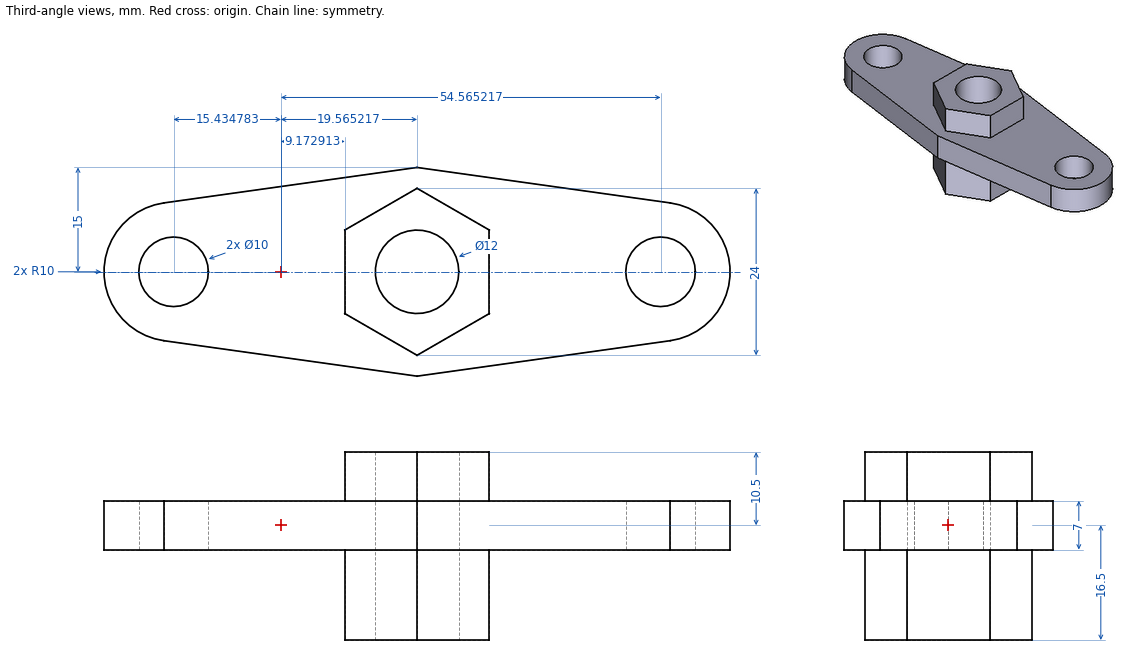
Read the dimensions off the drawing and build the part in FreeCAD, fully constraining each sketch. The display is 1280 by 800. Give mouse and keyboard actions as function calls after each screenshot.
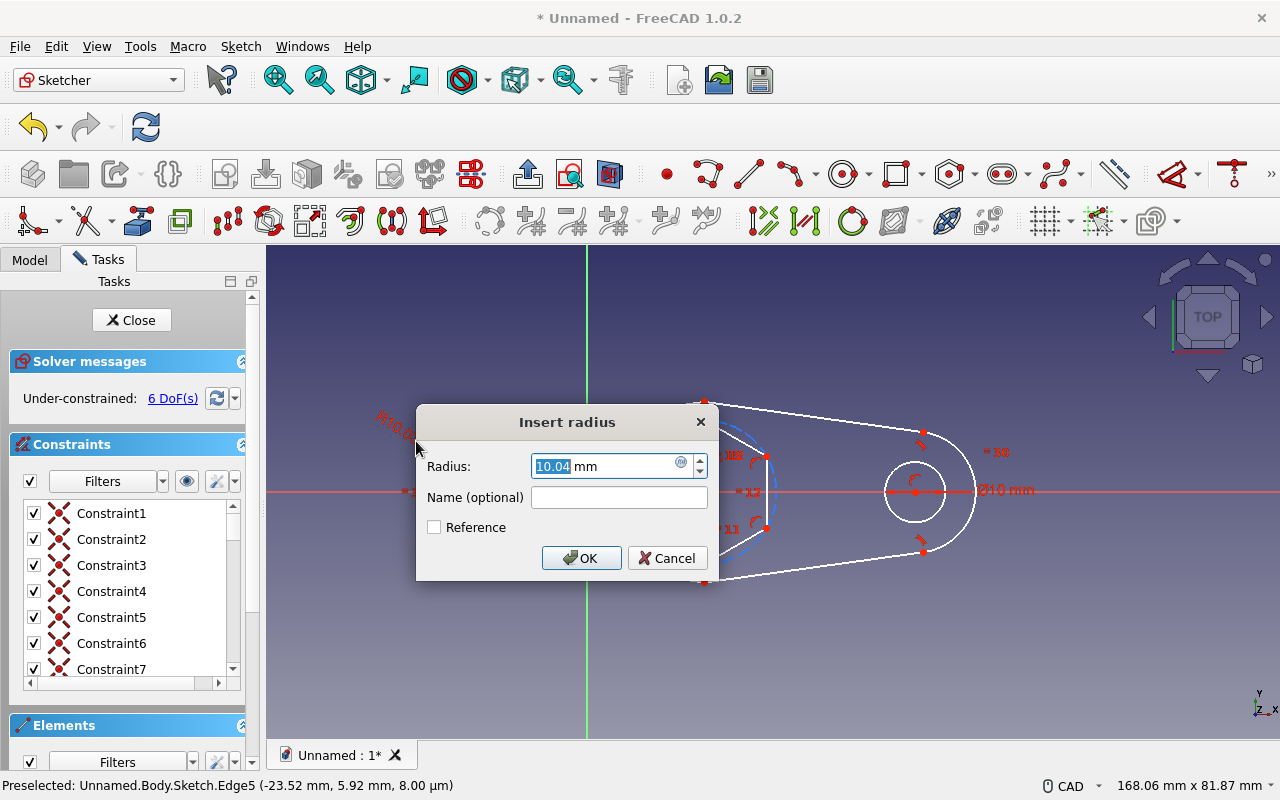
text(10)
key(Return)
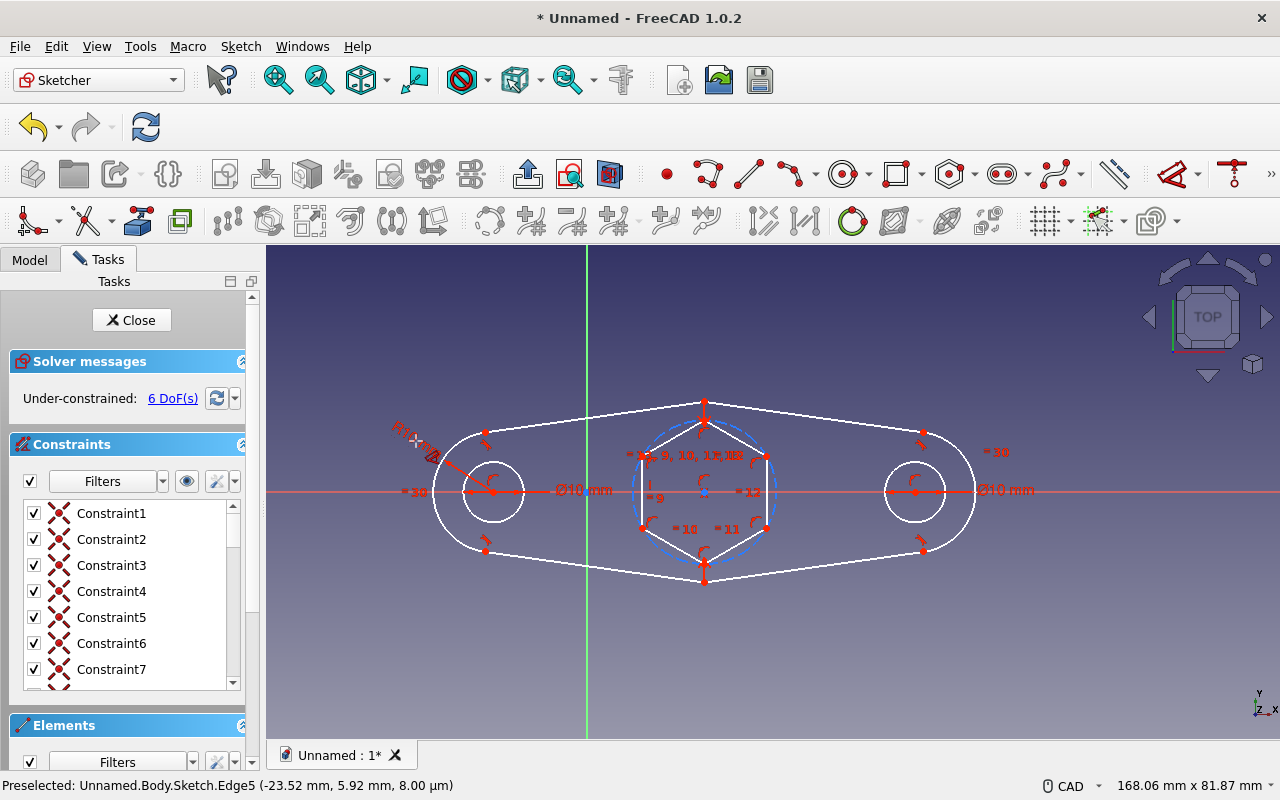
click(704, 564)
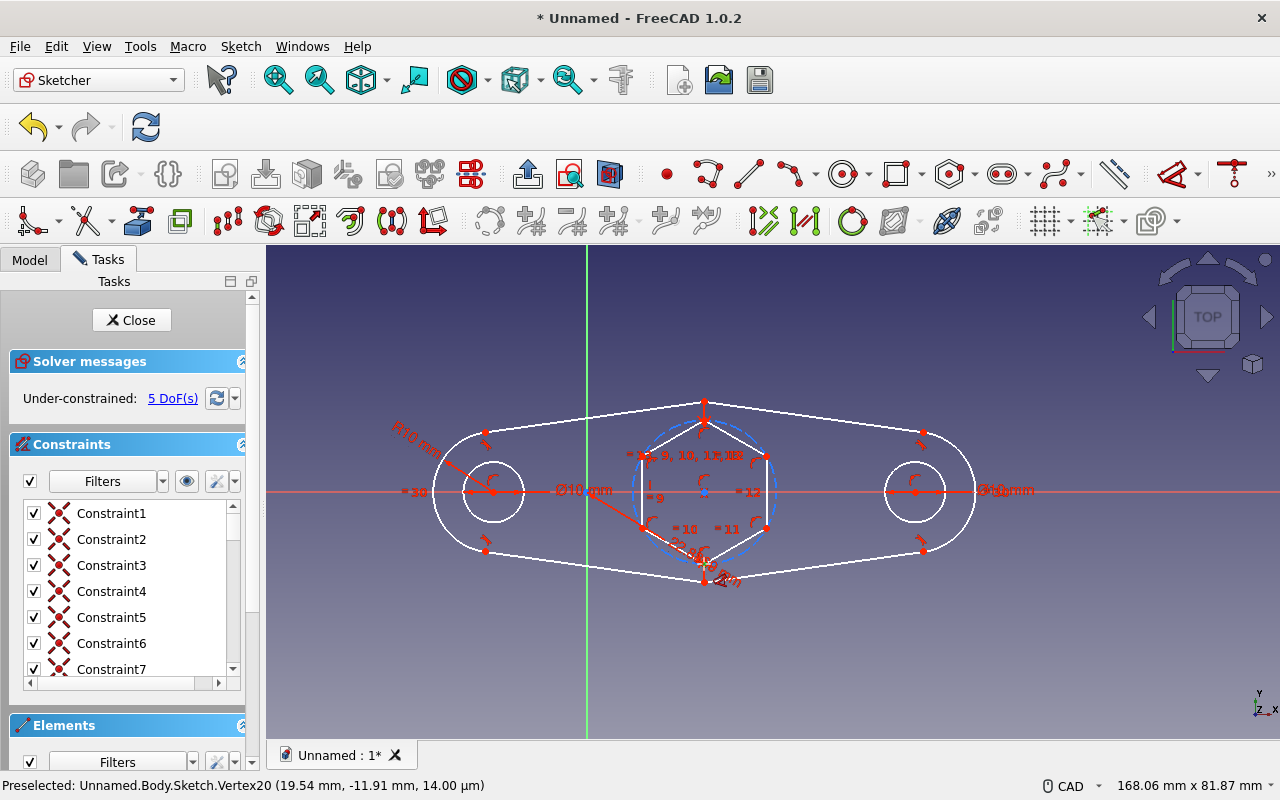
click(704, 420)
click(670, 459)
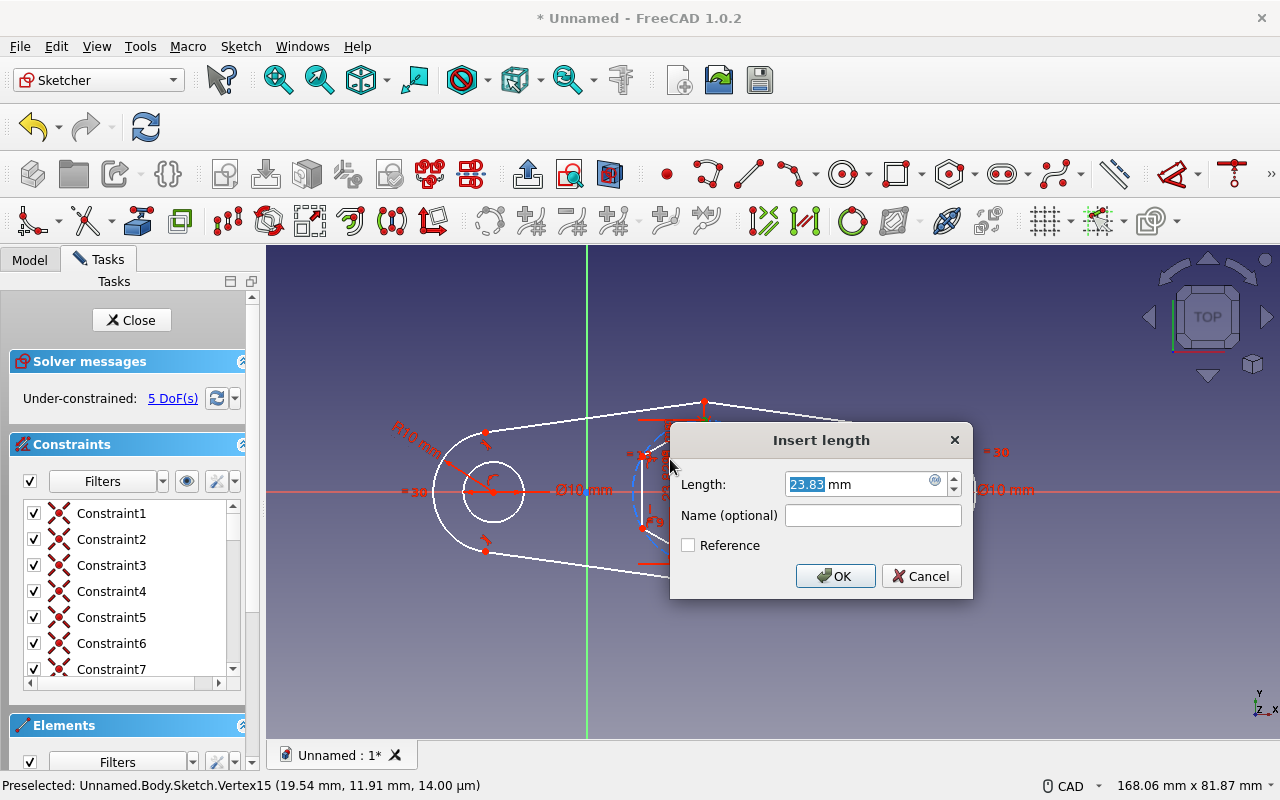
text(24)
key(Return)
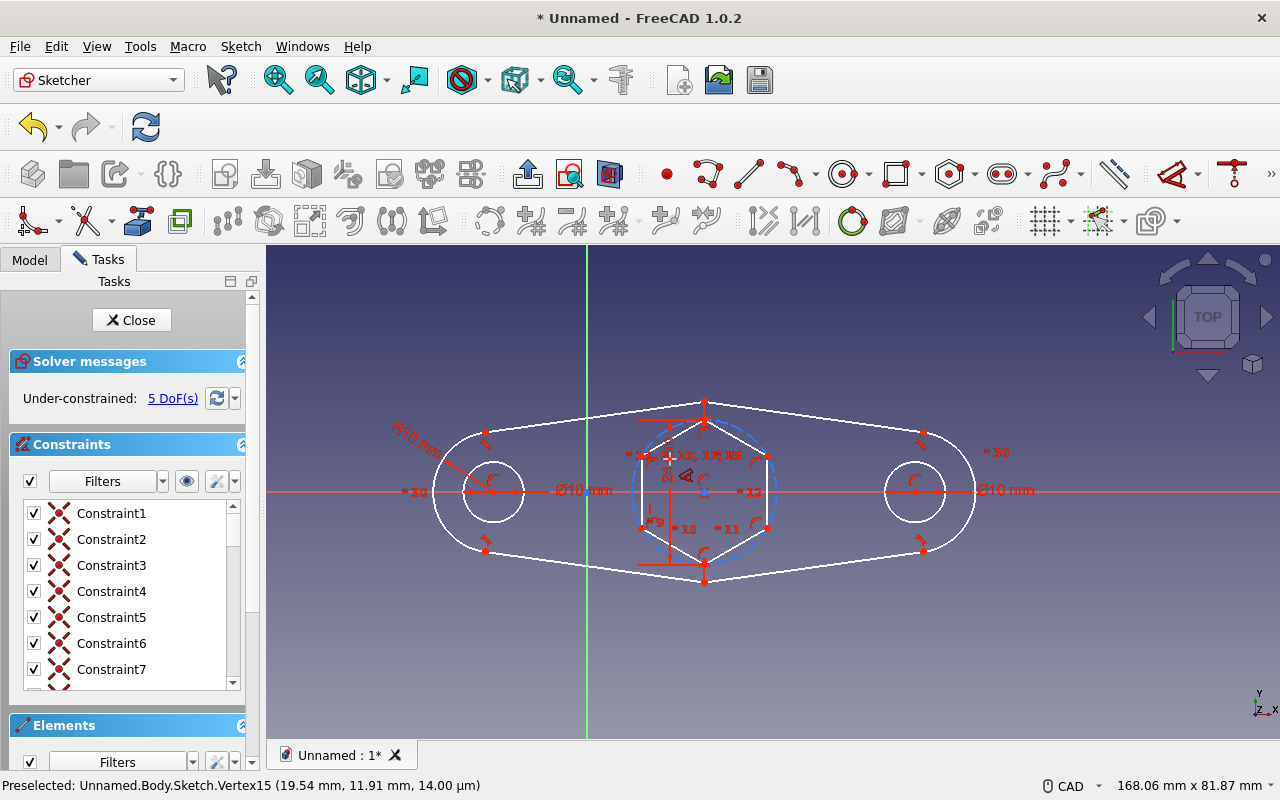
click(704, 402)
click(553, 447)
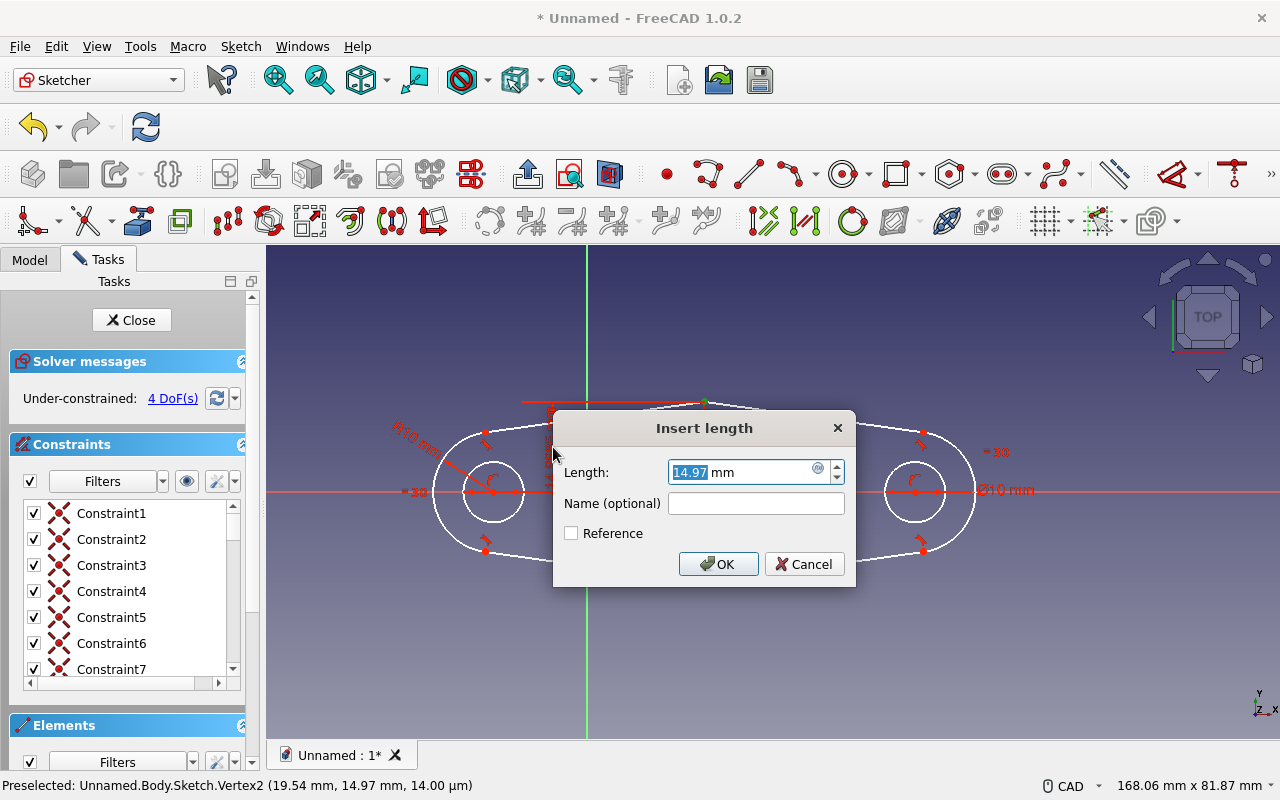
text(15)
key(Return)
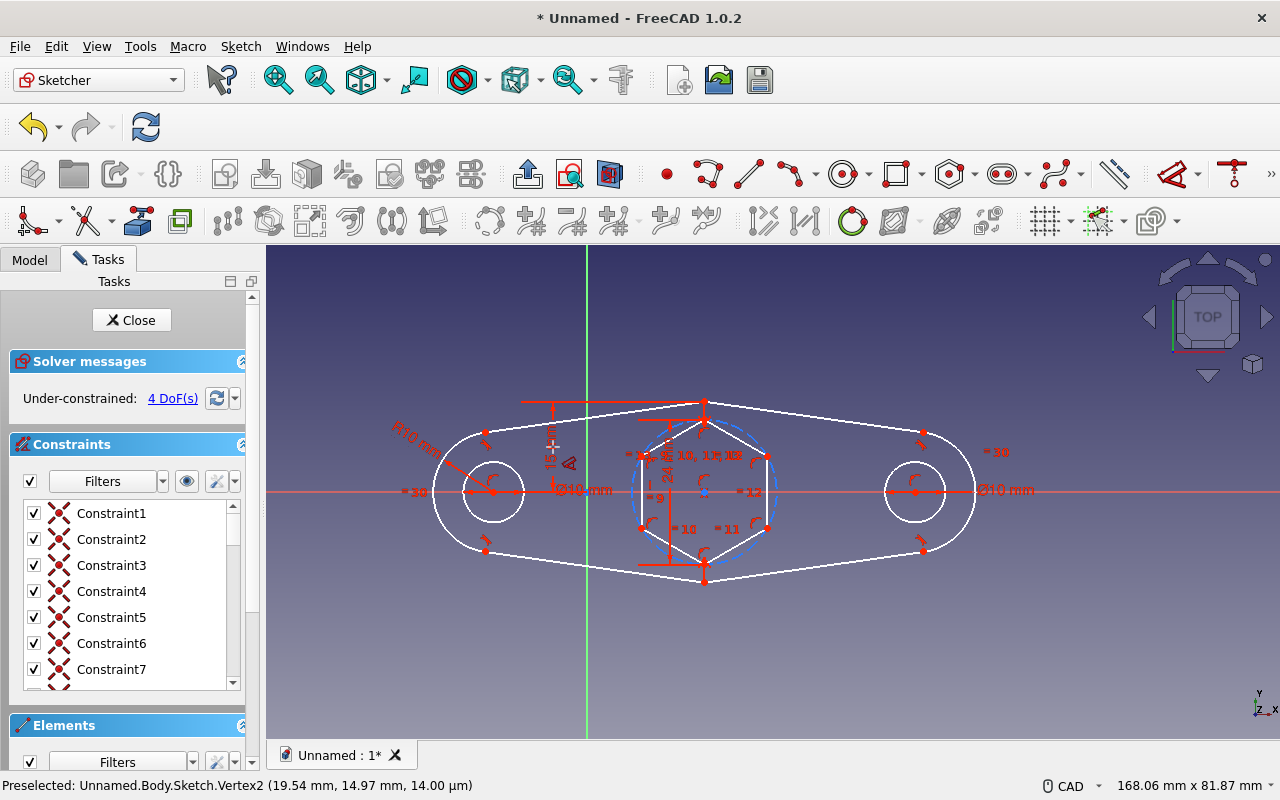
click(642, 456)
click(614, 526)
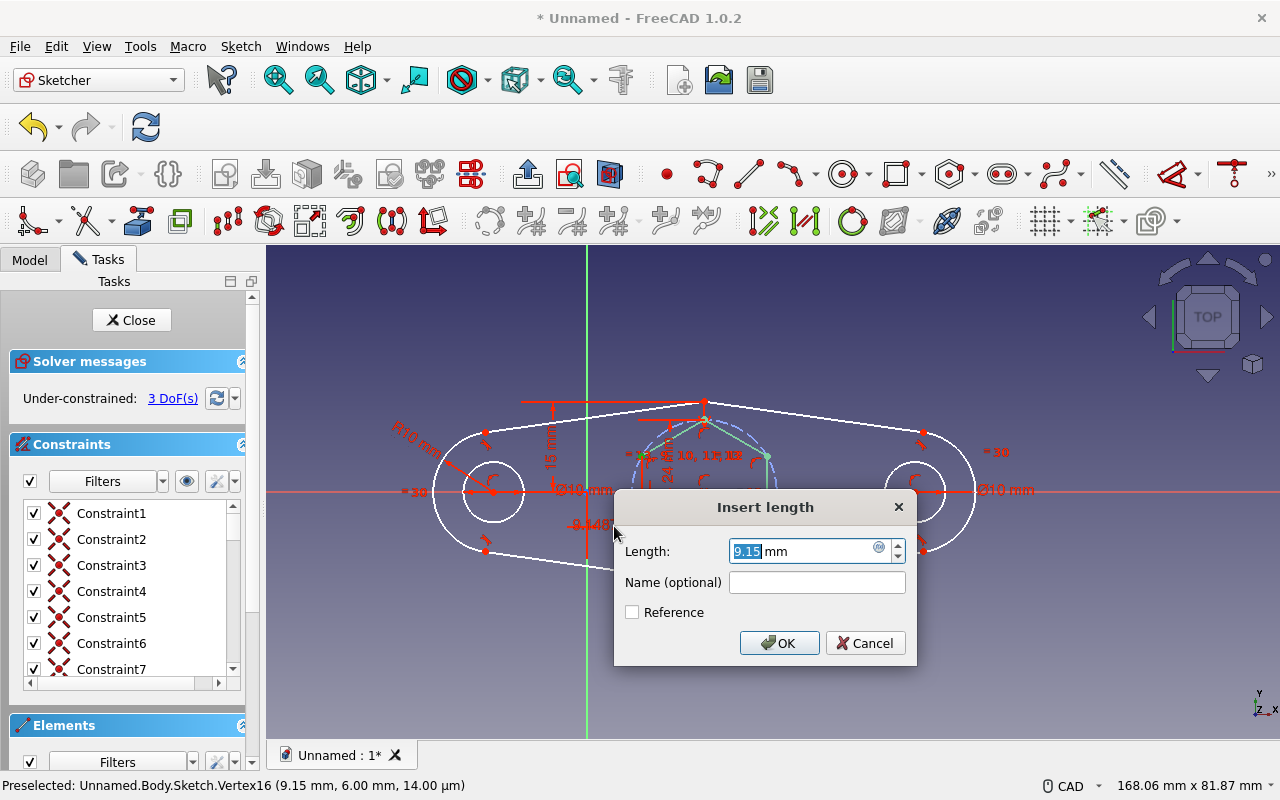
text(9.172913)
key(Return)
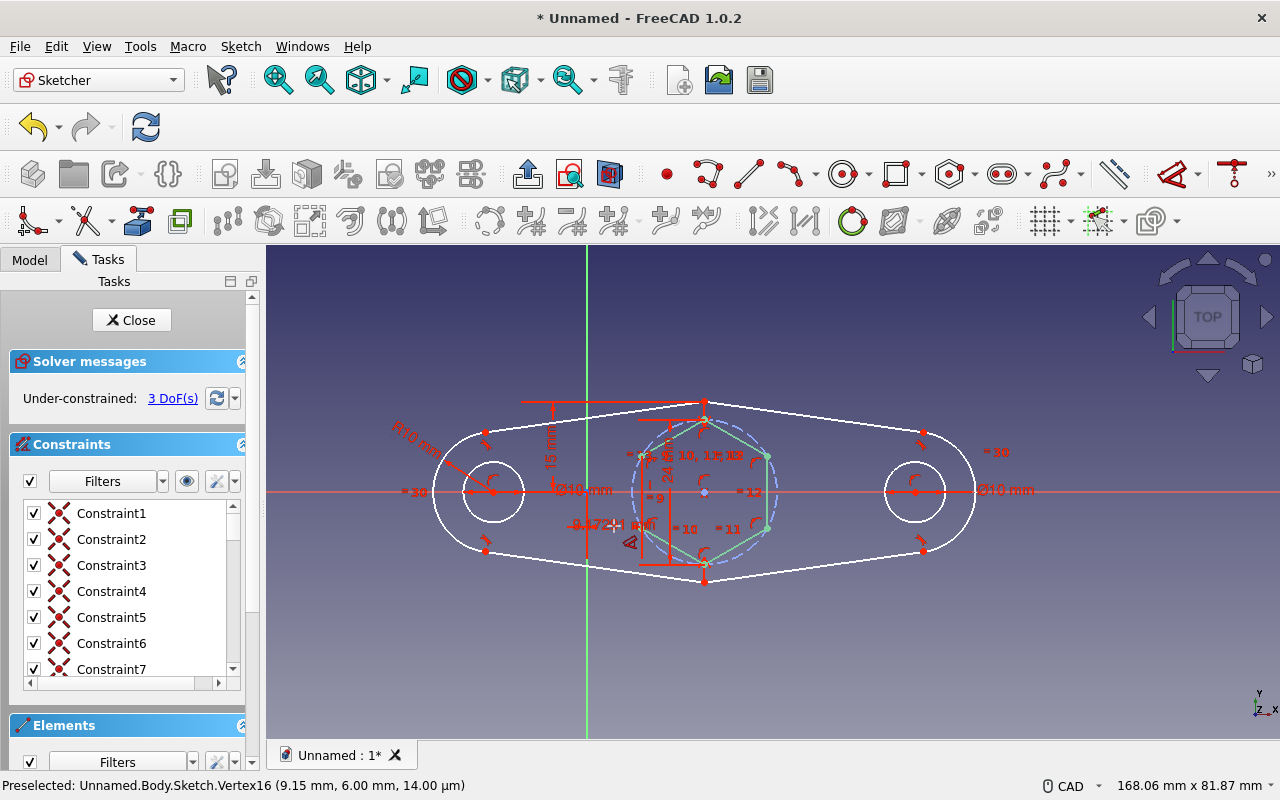
click(494, 492)
click(540, 526)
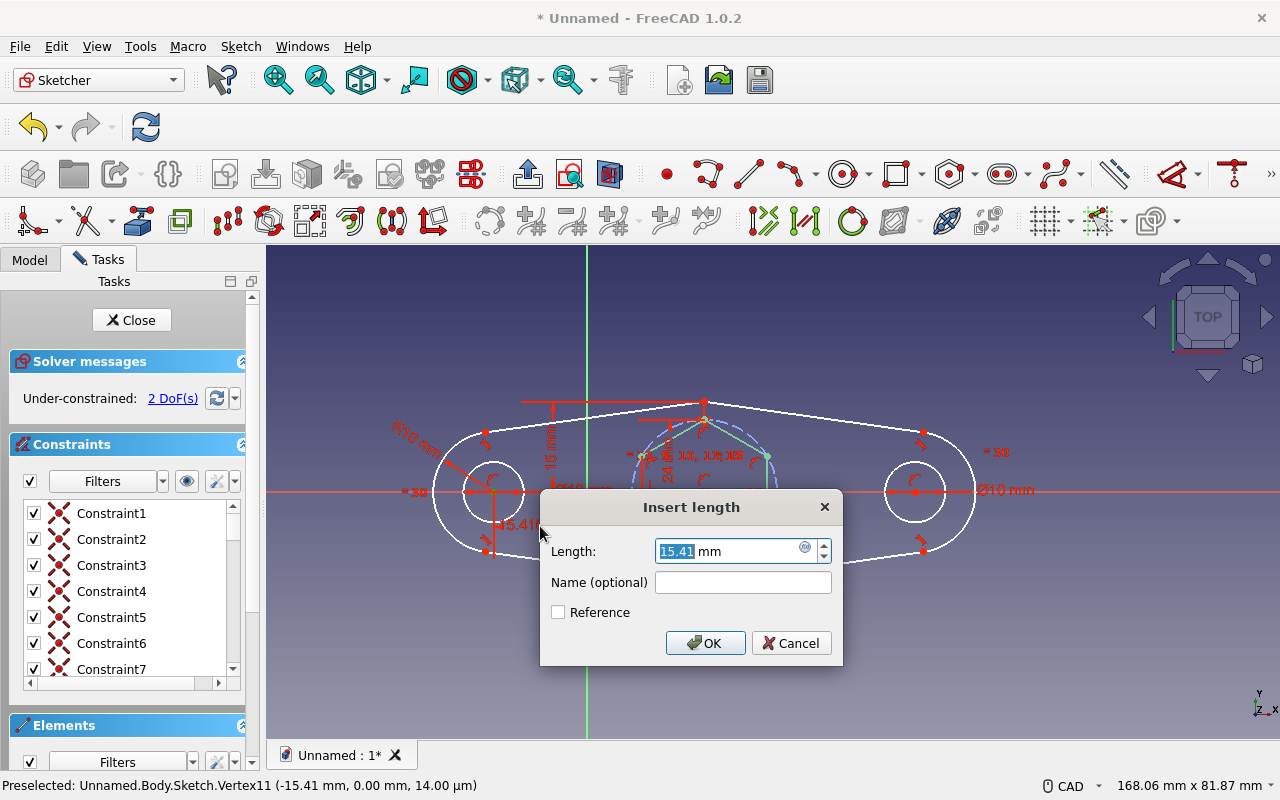
text(15.434783)
key(Return)